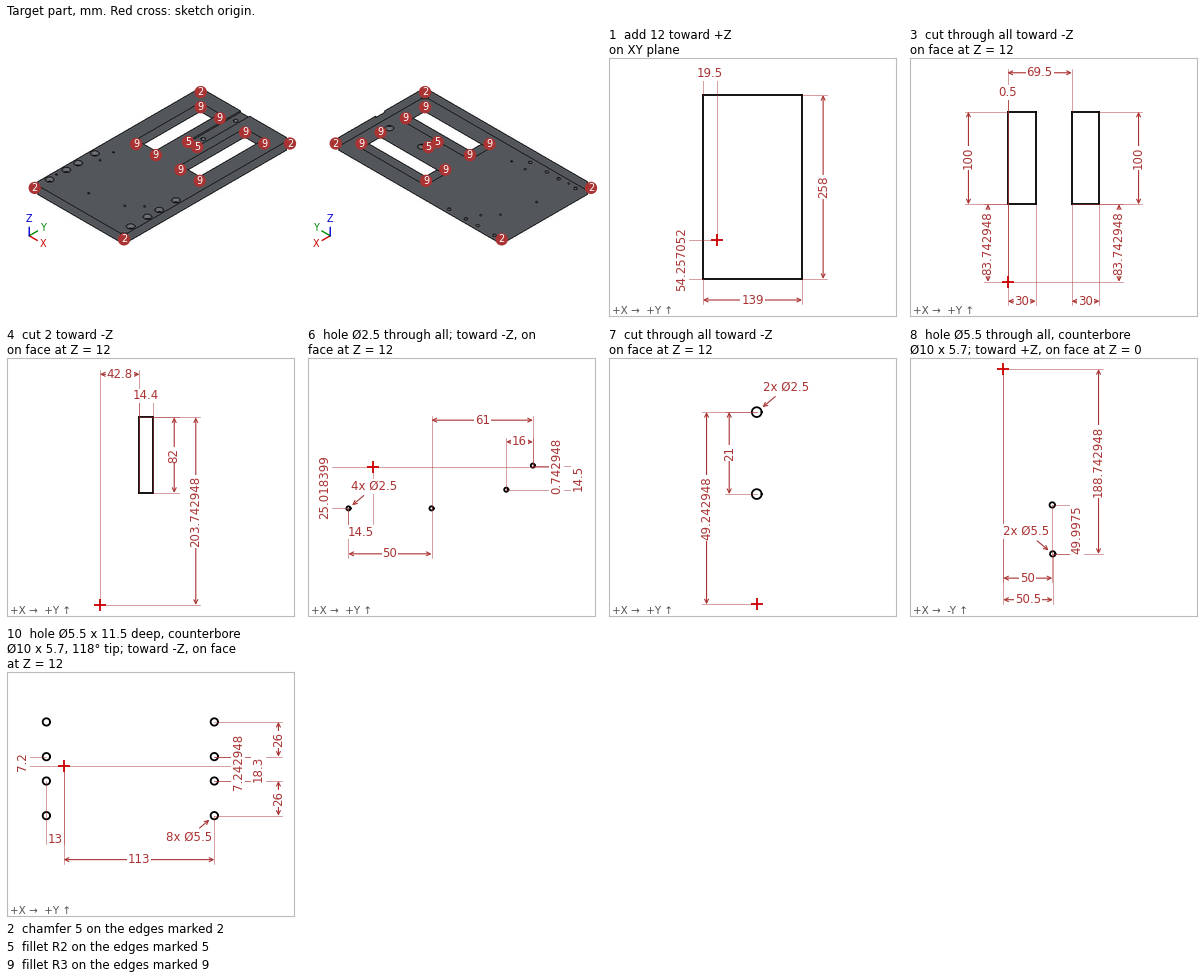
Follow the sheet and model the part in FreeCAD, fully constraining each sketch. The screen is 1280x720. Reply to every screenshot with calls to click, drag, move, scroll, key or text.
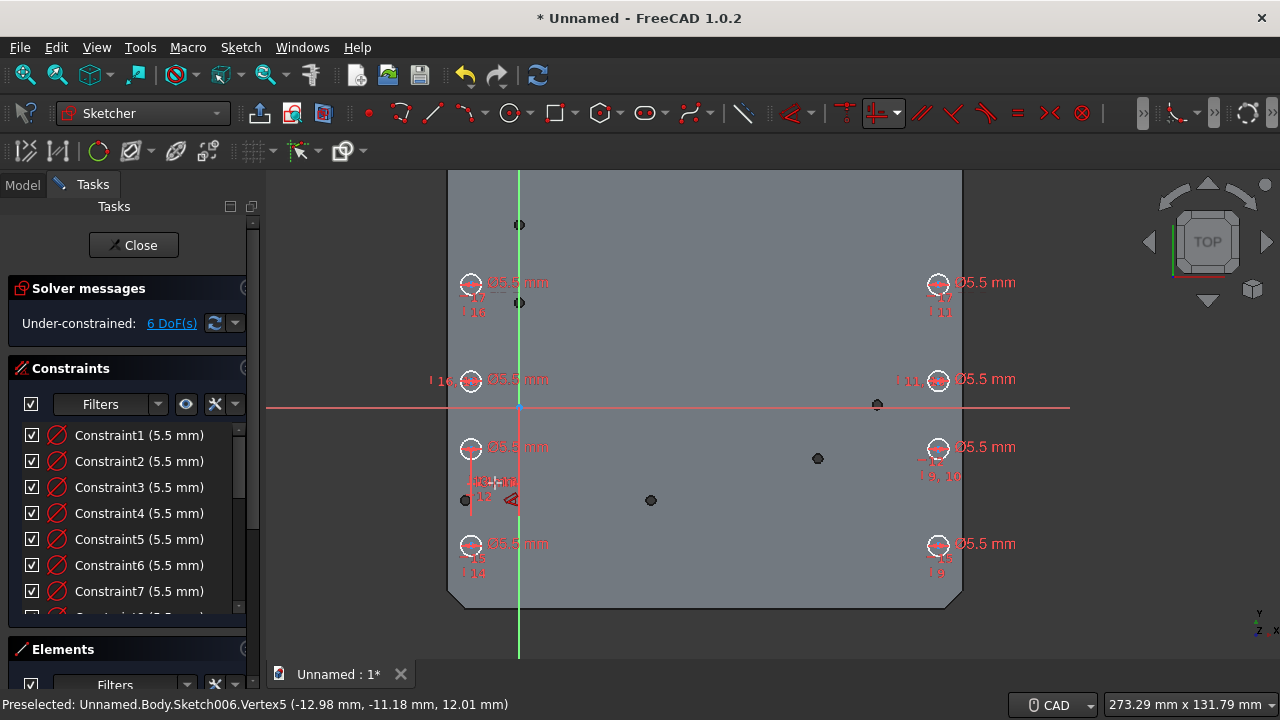
click(938, 546)
click(729, 580)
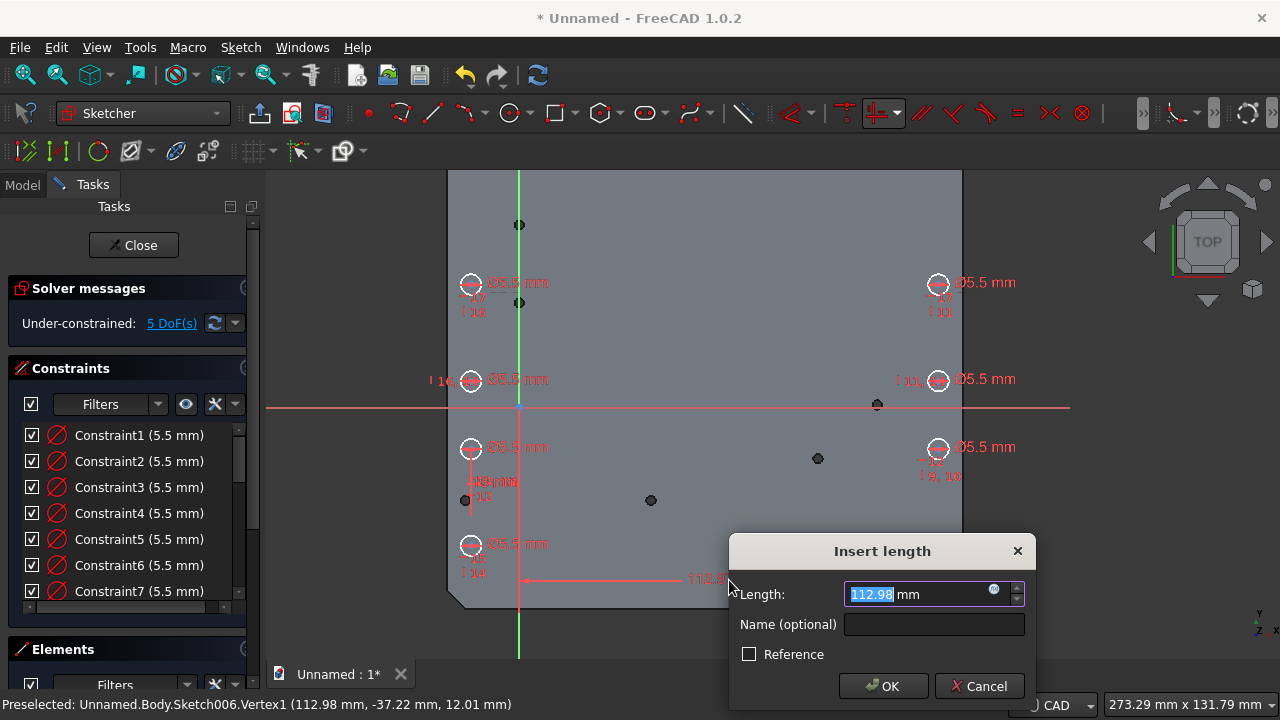
text(113)
key(Return)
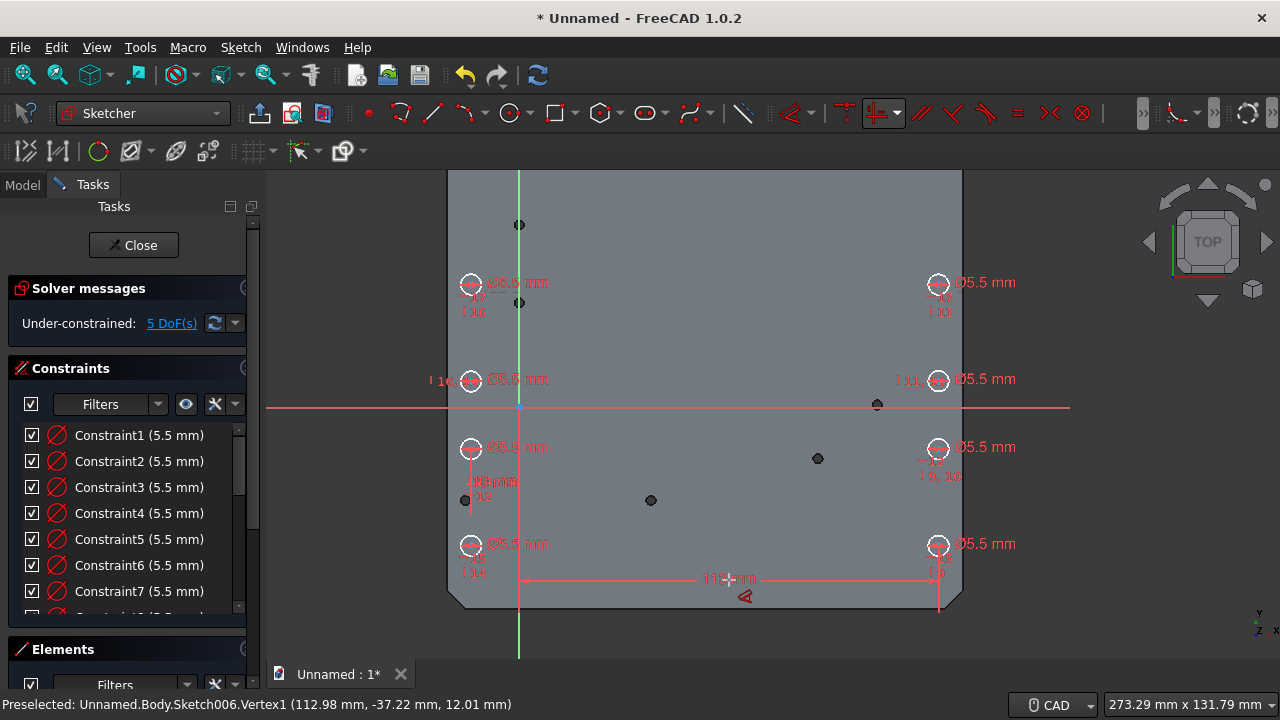
scroll(471, 381, up, 2)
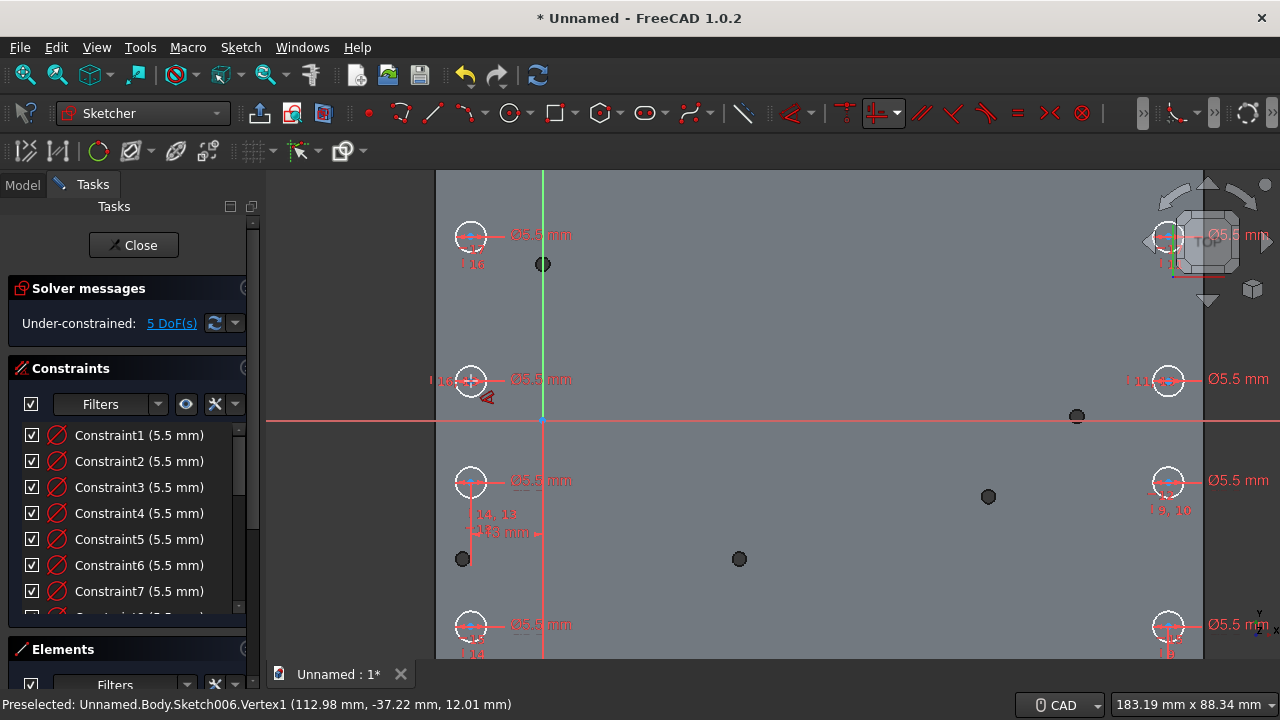
click(471, 381)
click(437, 401)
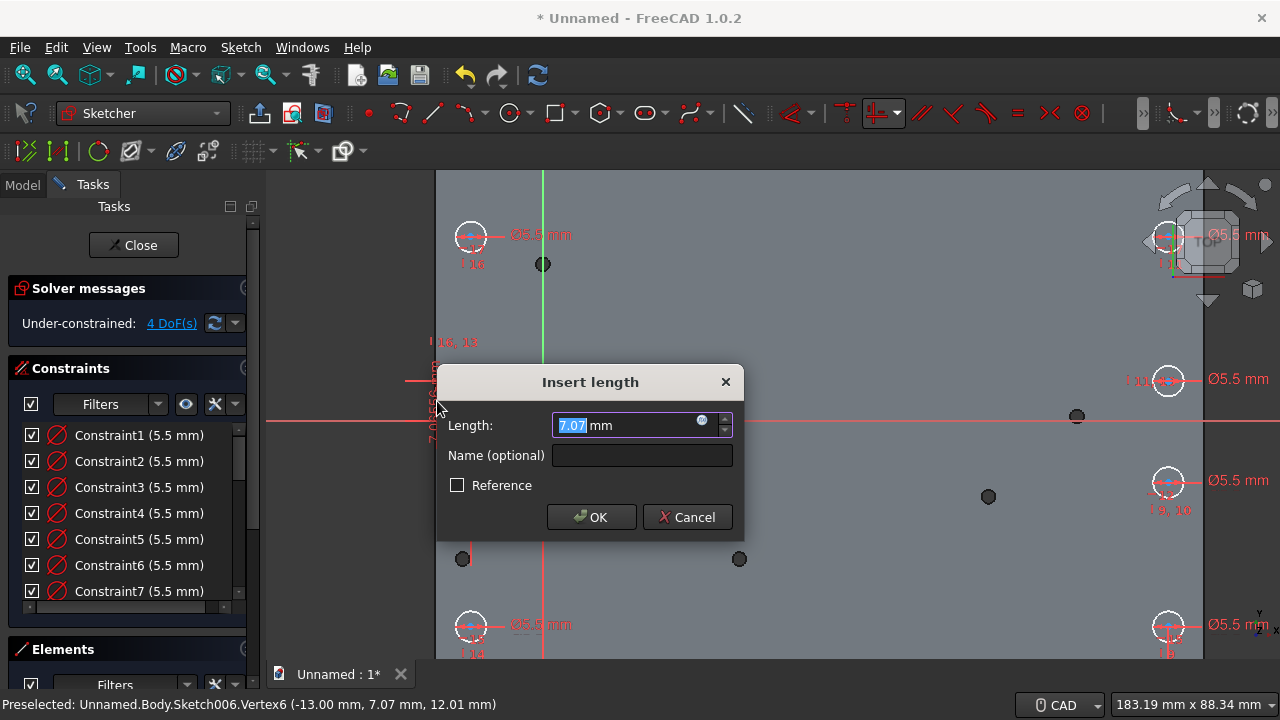
text(7.2)
key(Return)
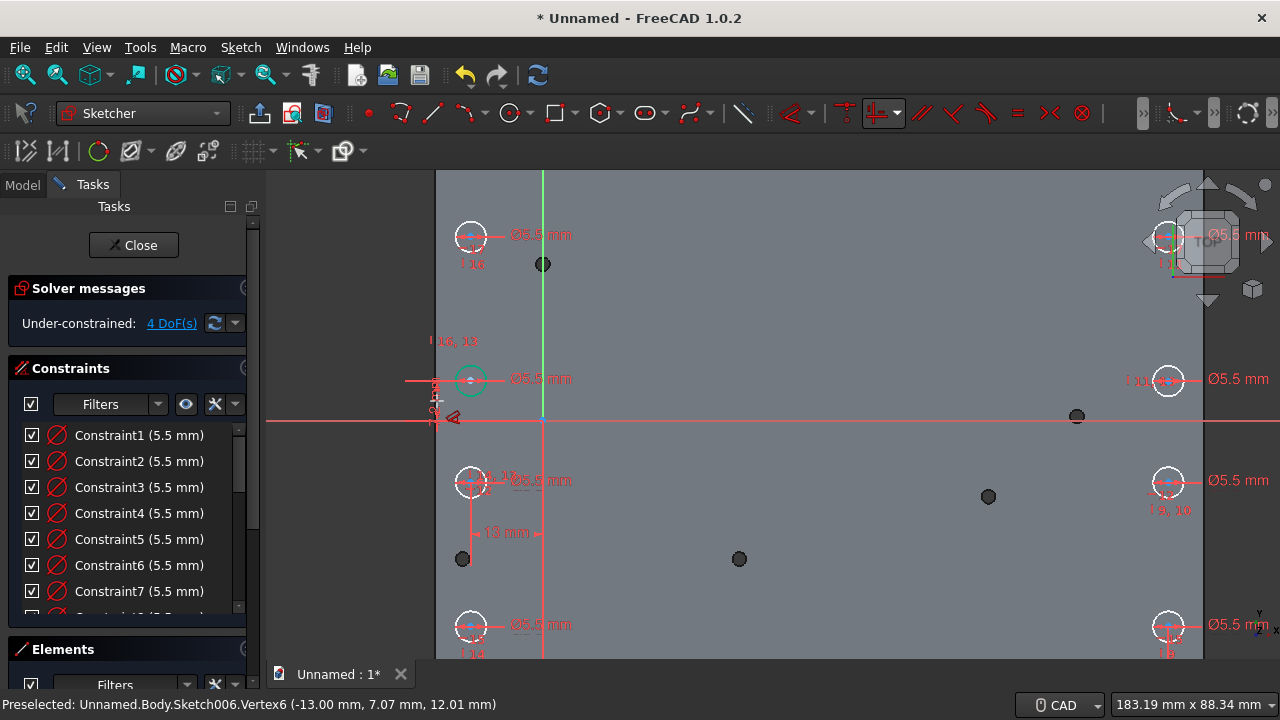
scroll(470, 381, down, 2)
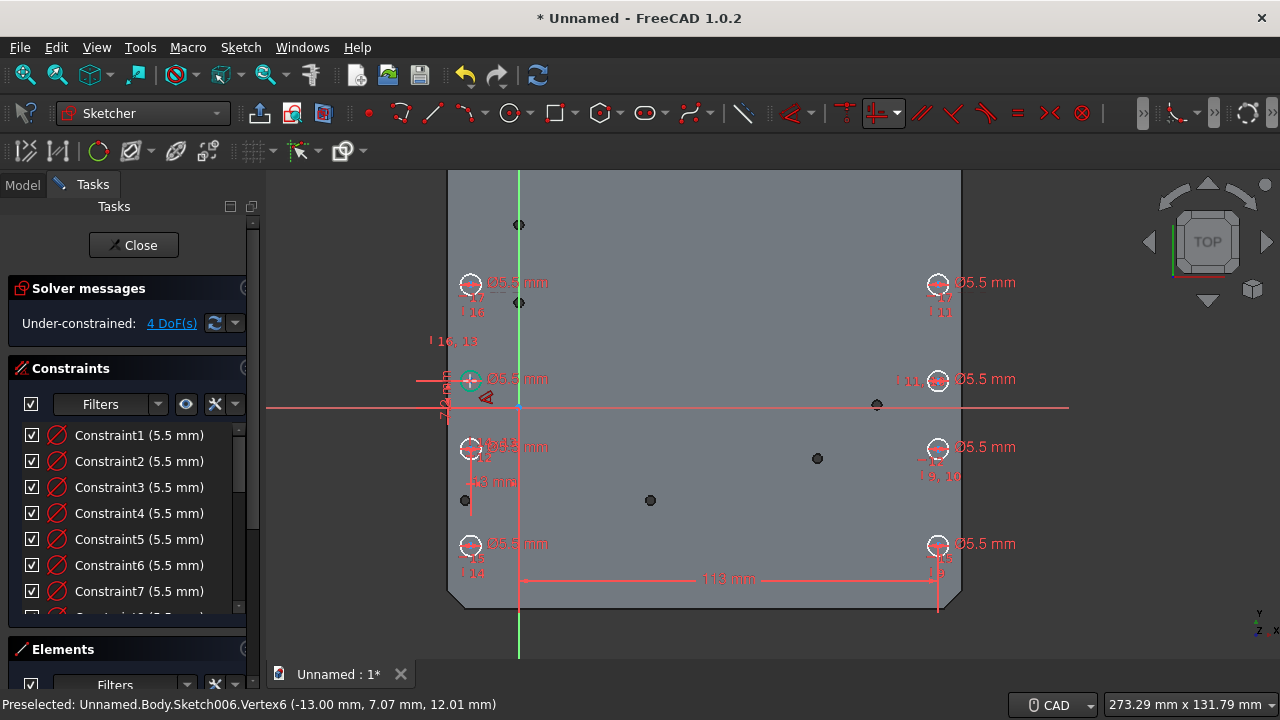
click(938, 546)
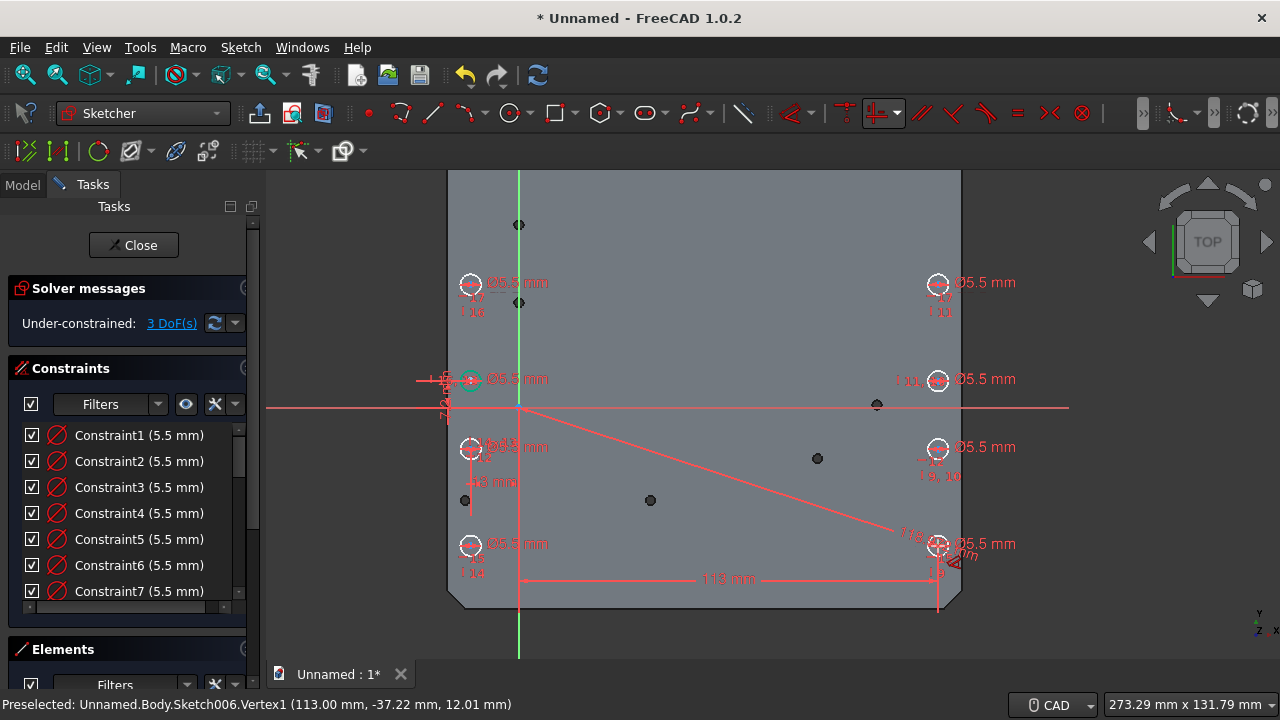
click(938, 449)
click(972, 497)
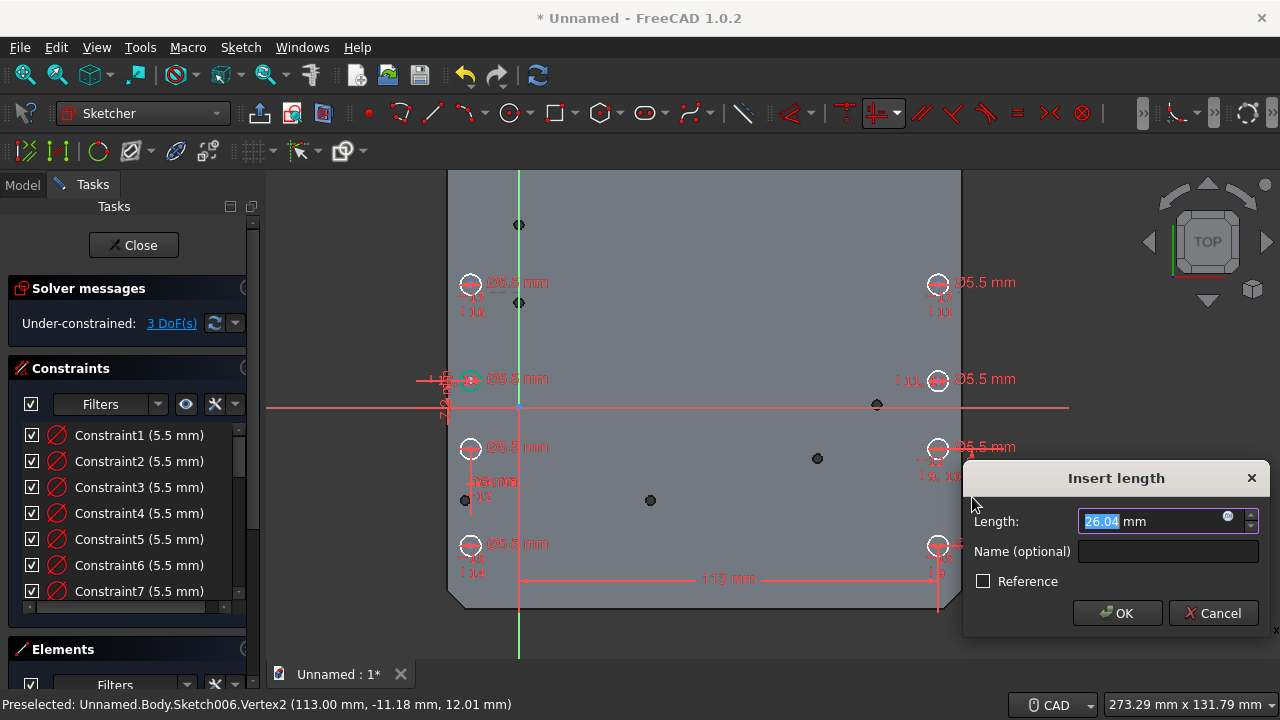
text(26)
key(Return)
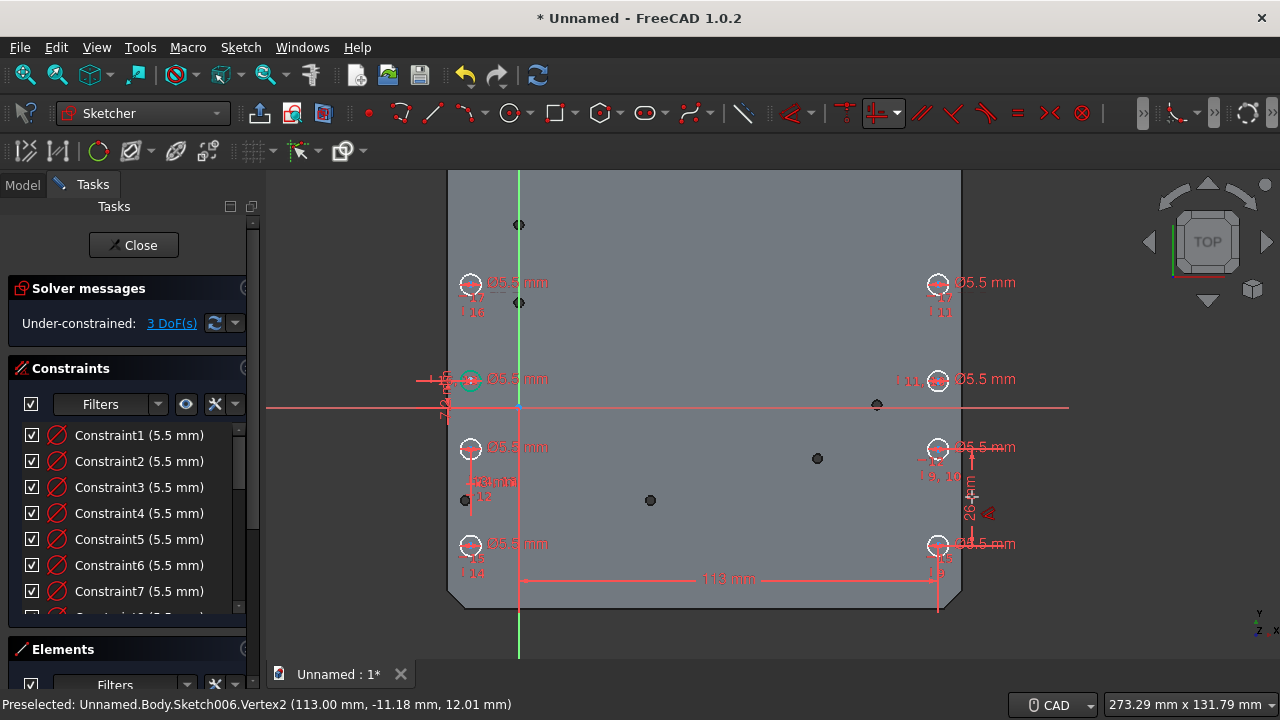
click(938, 381)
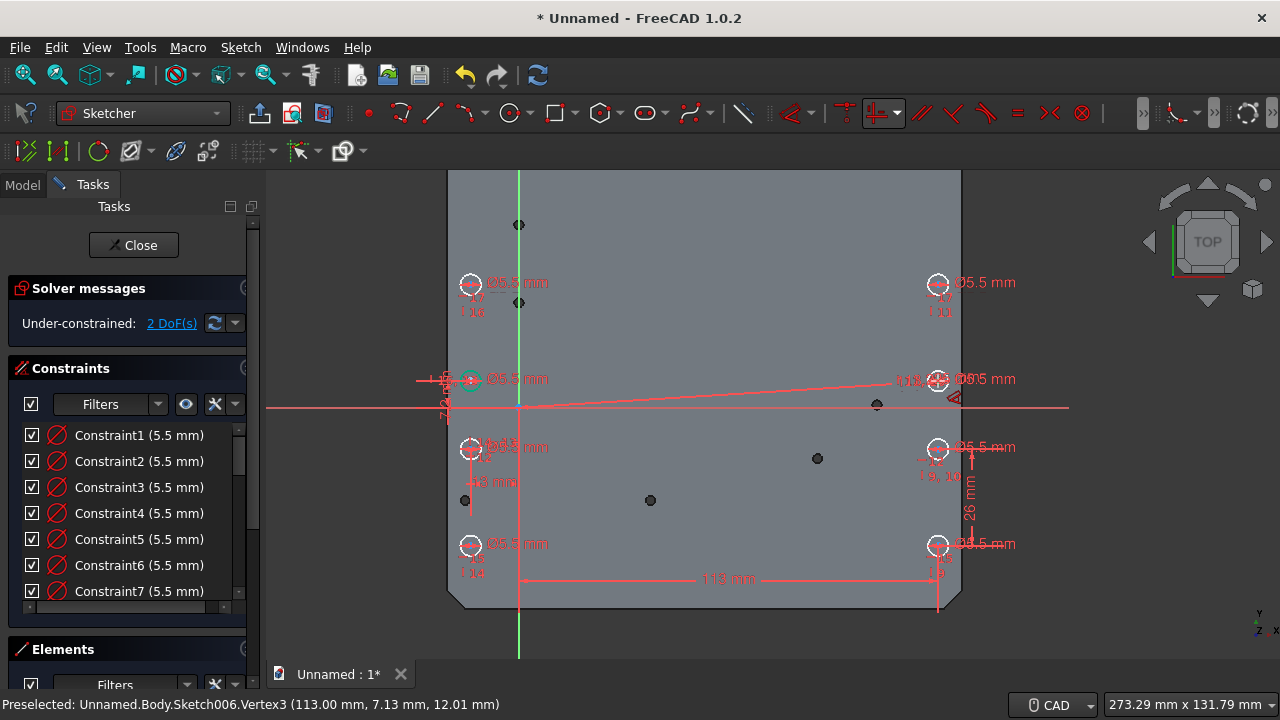
click(938, 285)
click(972, 333)